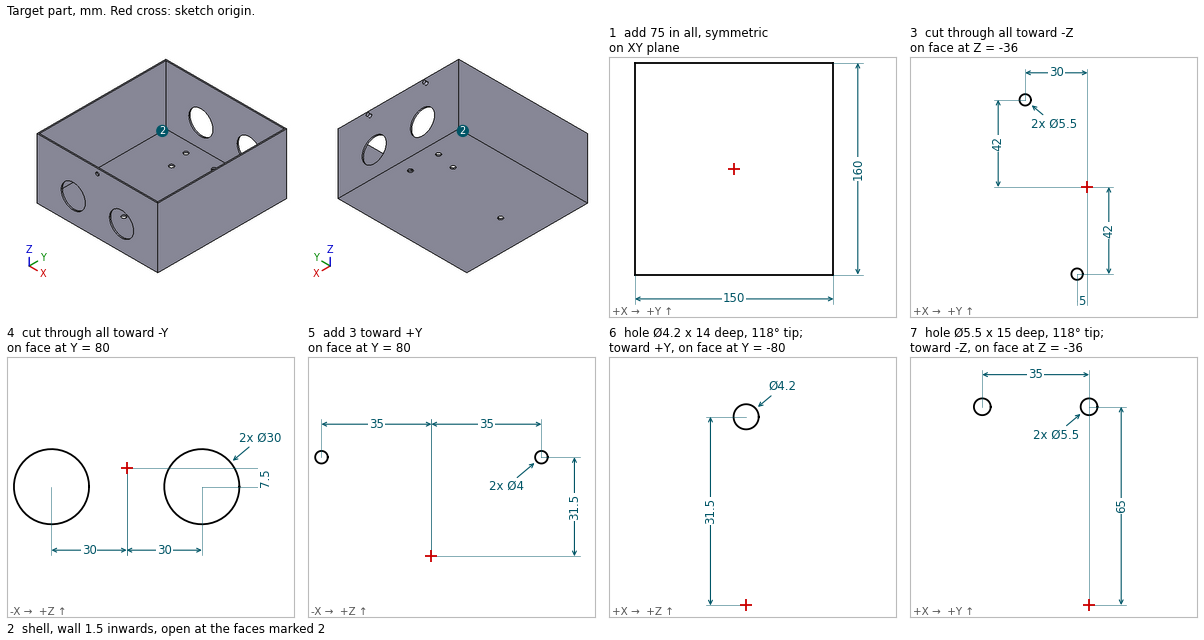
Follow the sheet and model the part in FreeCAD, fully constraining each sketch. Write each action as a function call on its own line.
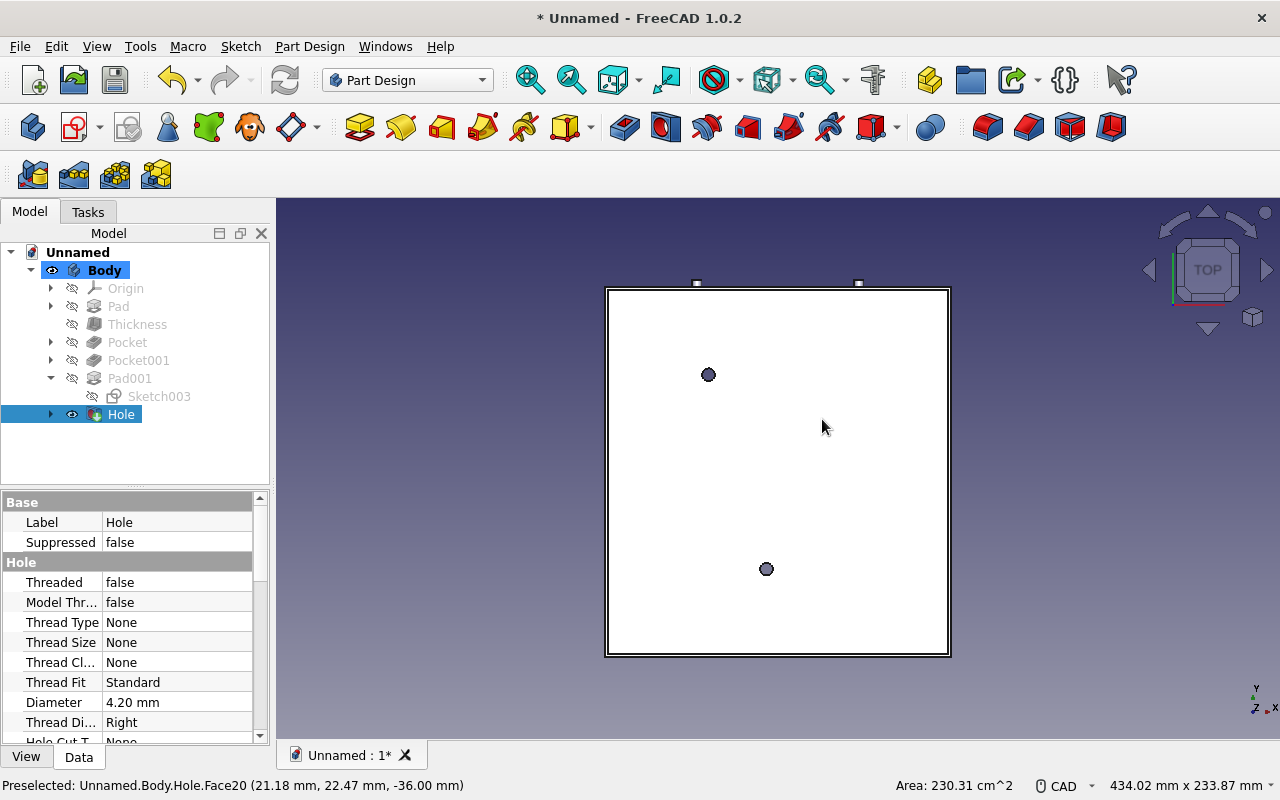
click(74, 128)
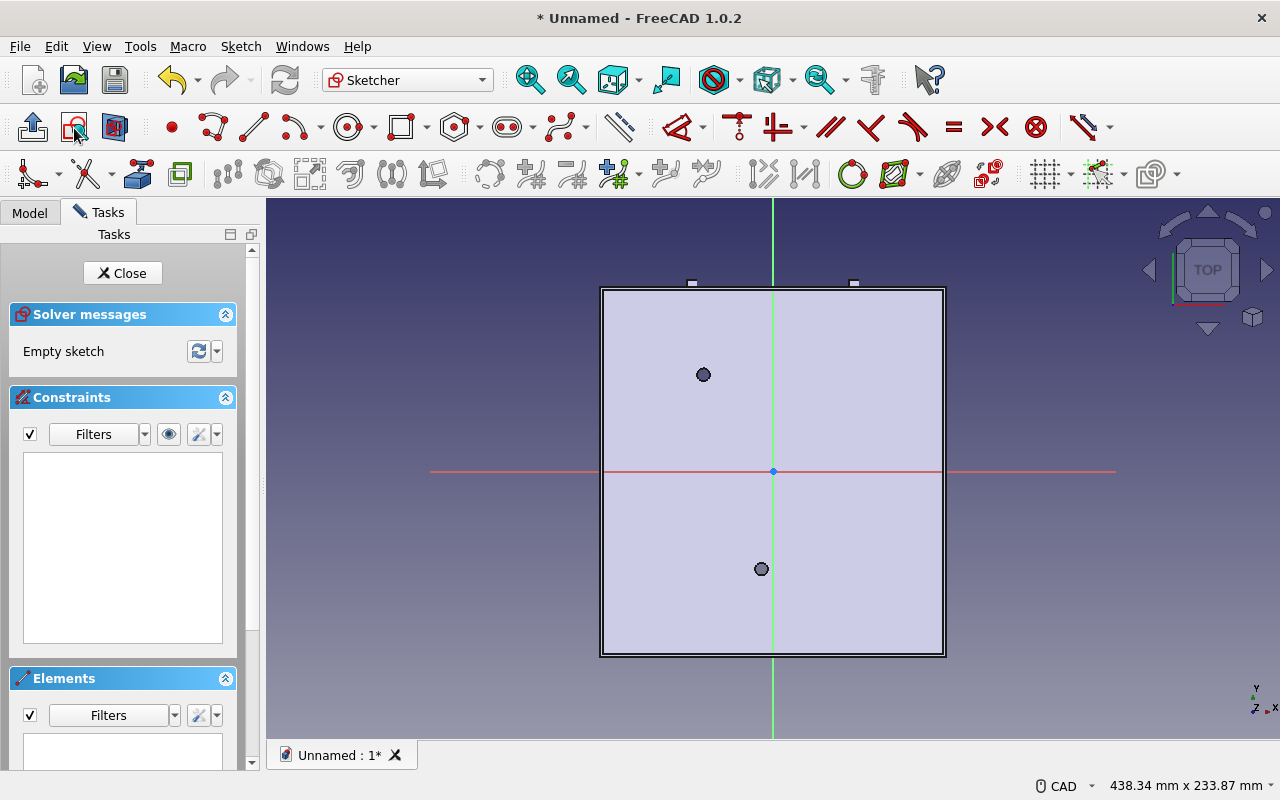
click(115, 128)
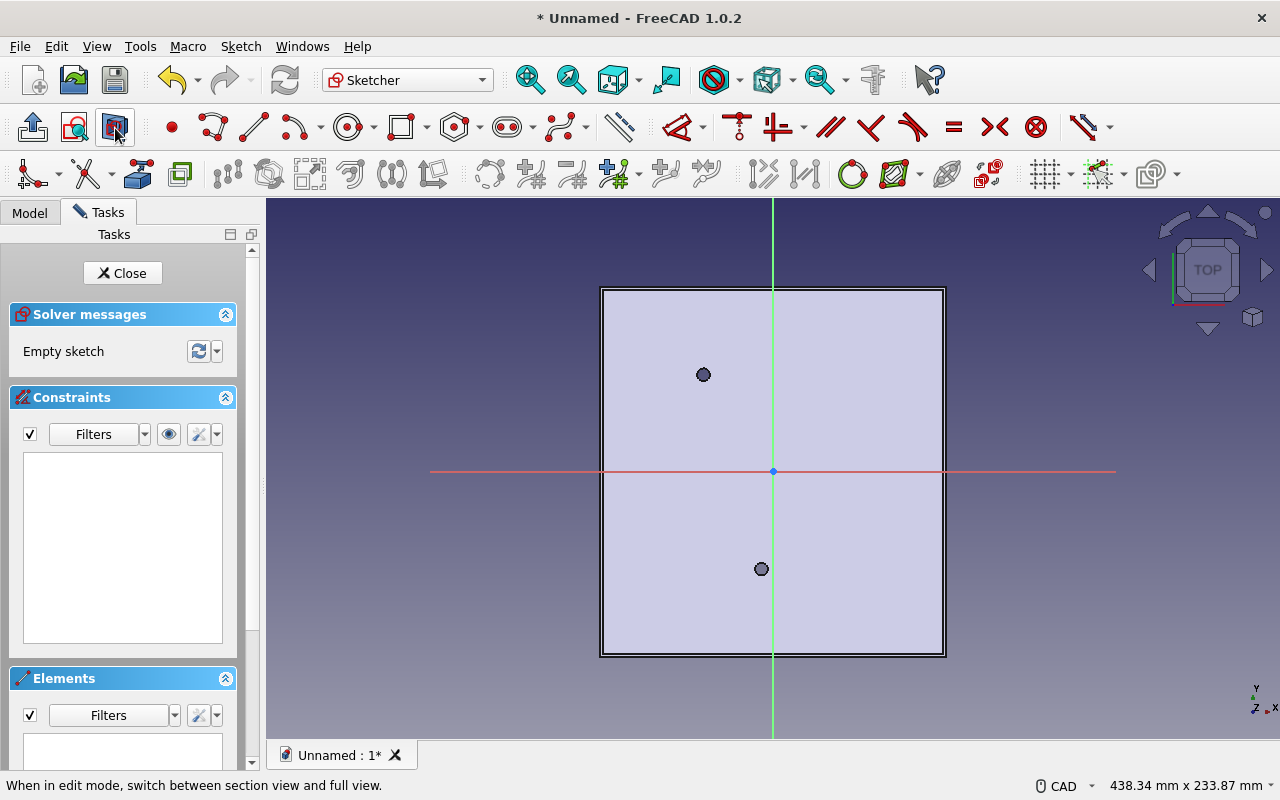
scroll(755, 332, up, 4)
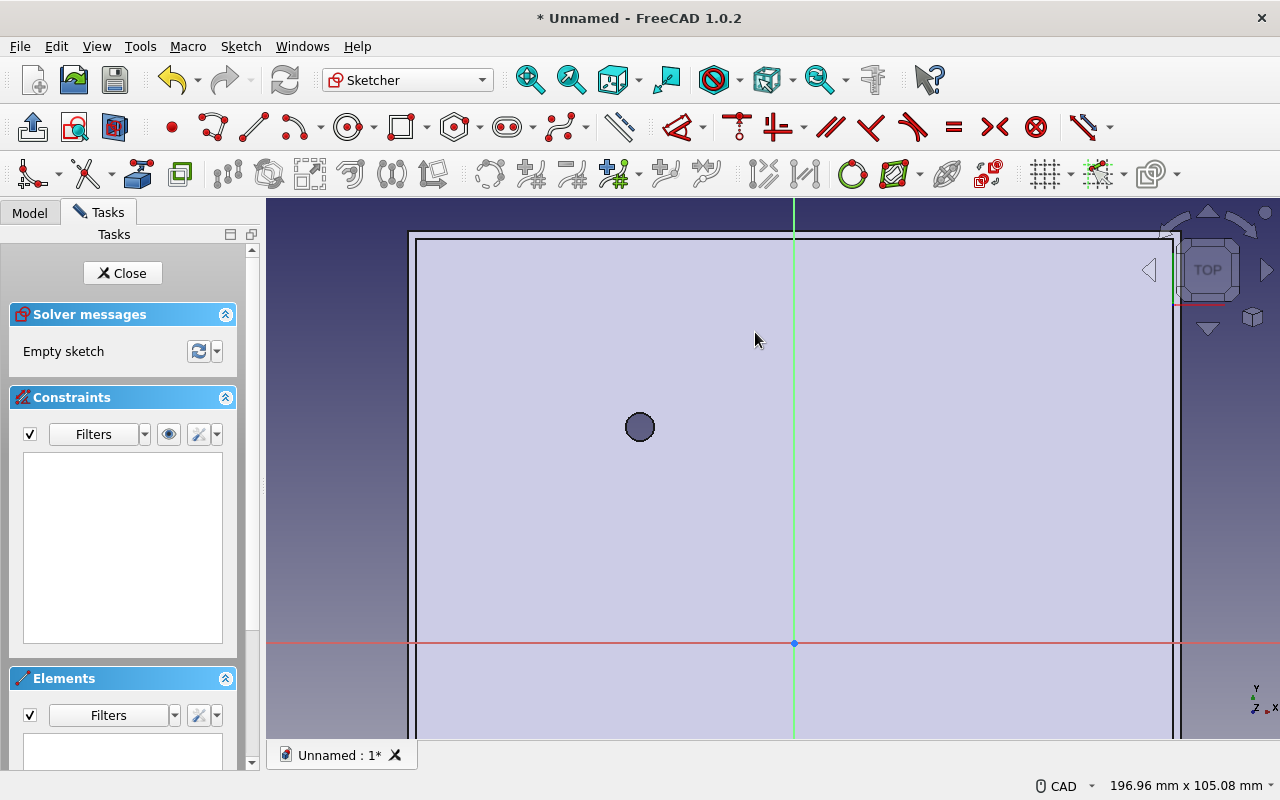
click(348, 128)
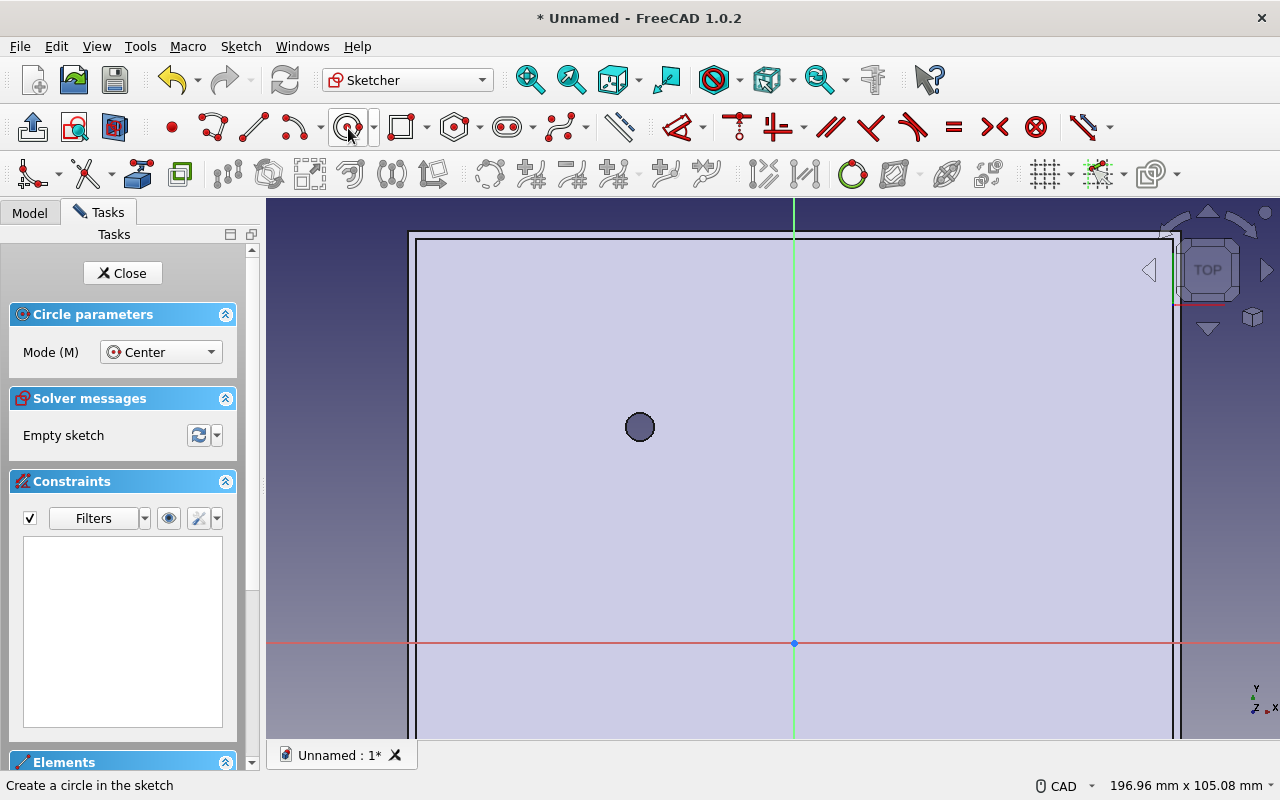
scroll(794, 309, up, 3)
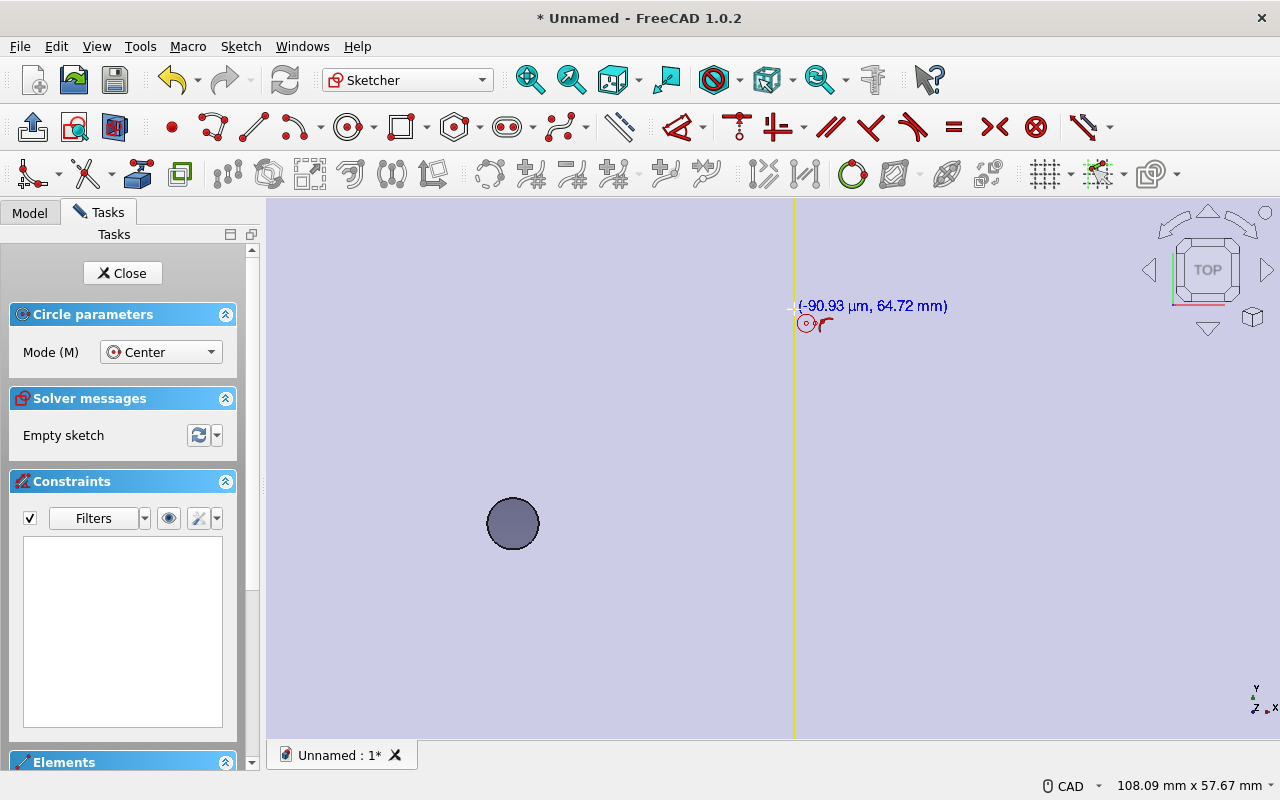
click(794, 308)
move(813, 290)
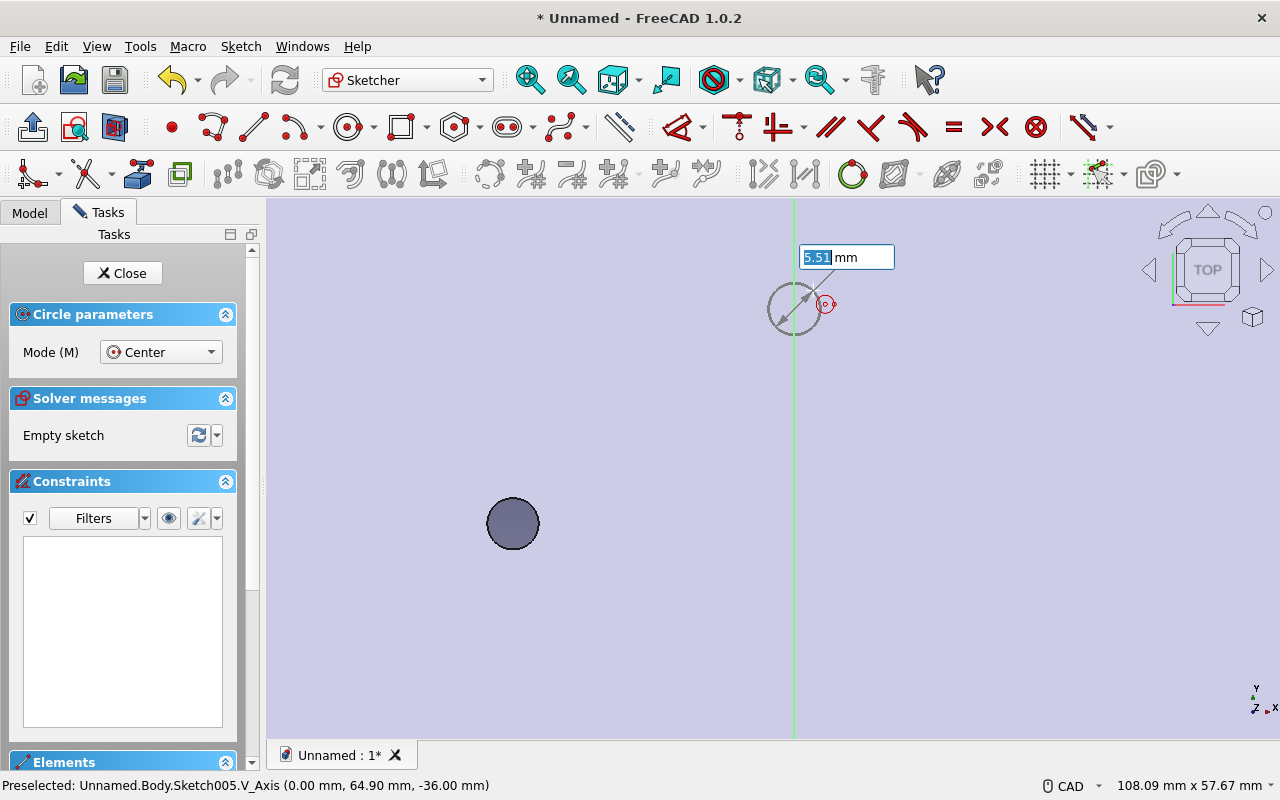
text(5.5)
key(Return)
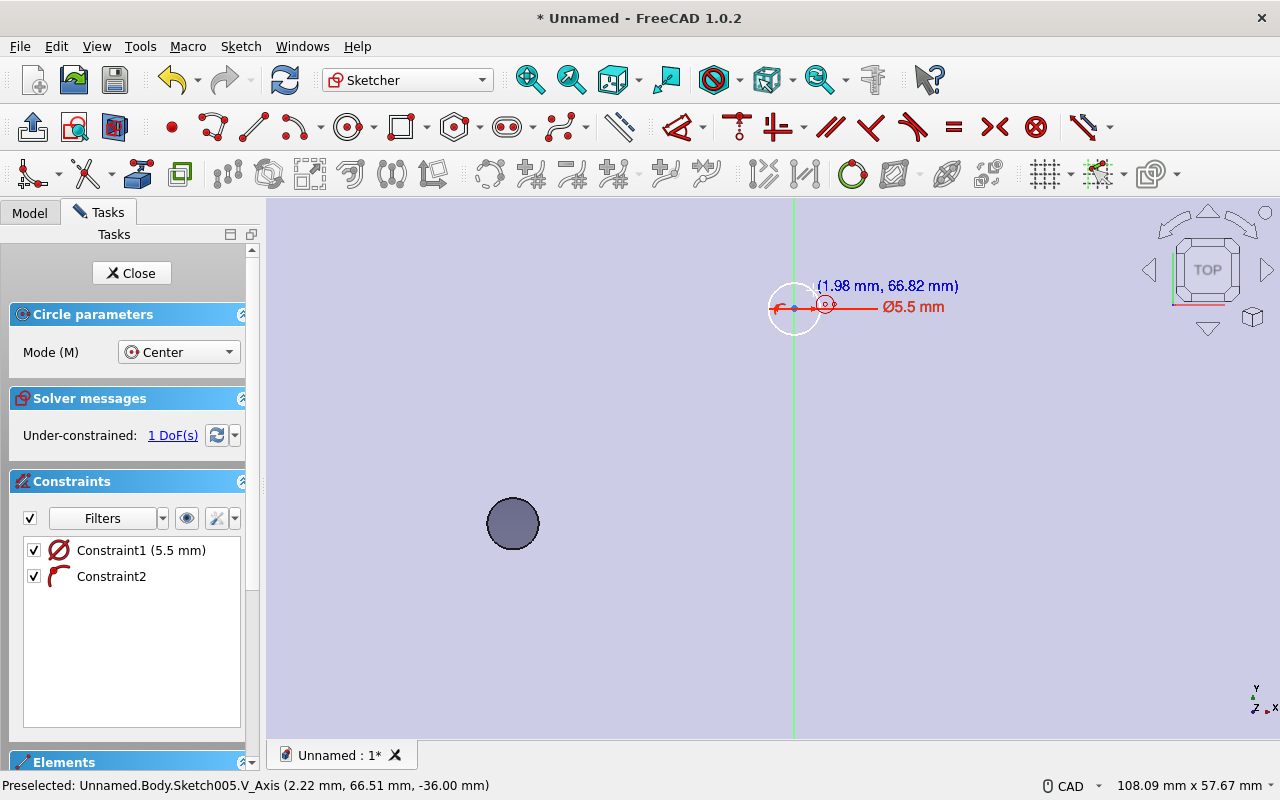
click(466, 308)
move(484, 290)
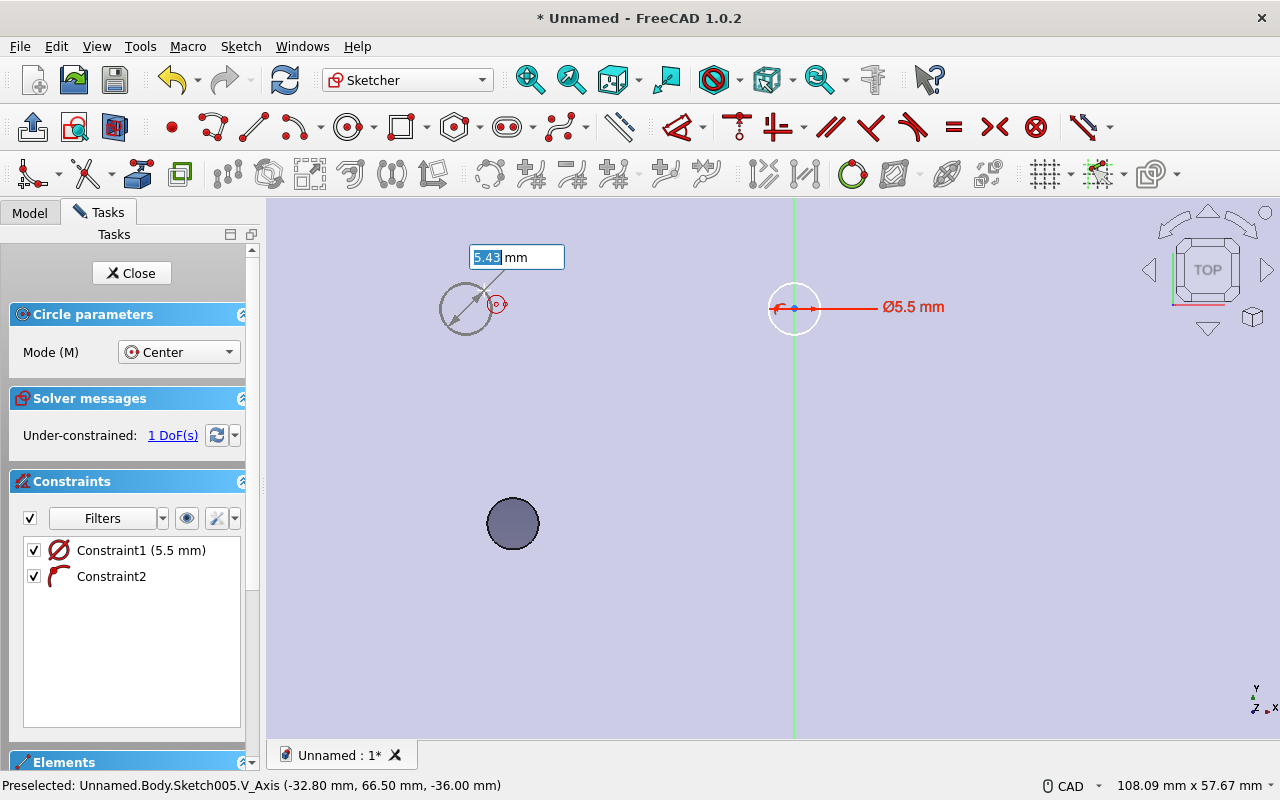
text(5.5)
key(Return)
key(Escape)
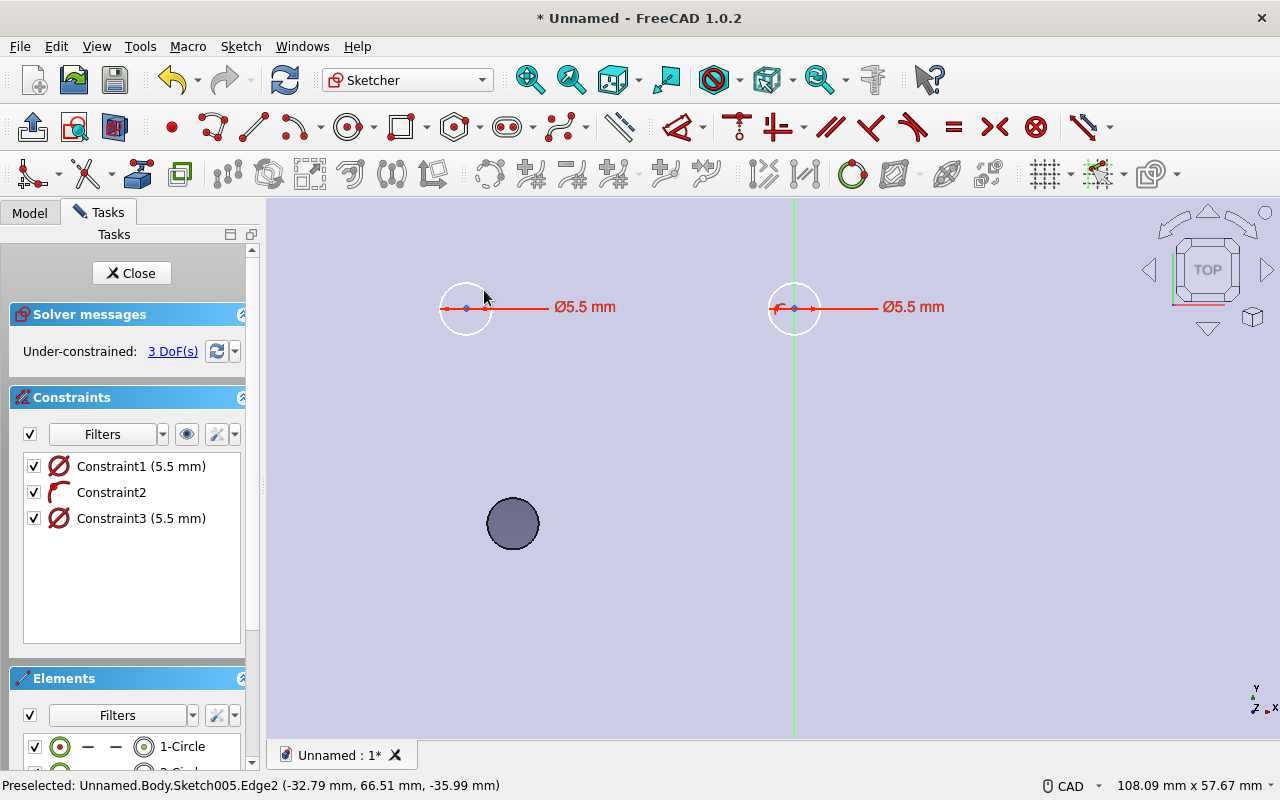
click(794, 309)